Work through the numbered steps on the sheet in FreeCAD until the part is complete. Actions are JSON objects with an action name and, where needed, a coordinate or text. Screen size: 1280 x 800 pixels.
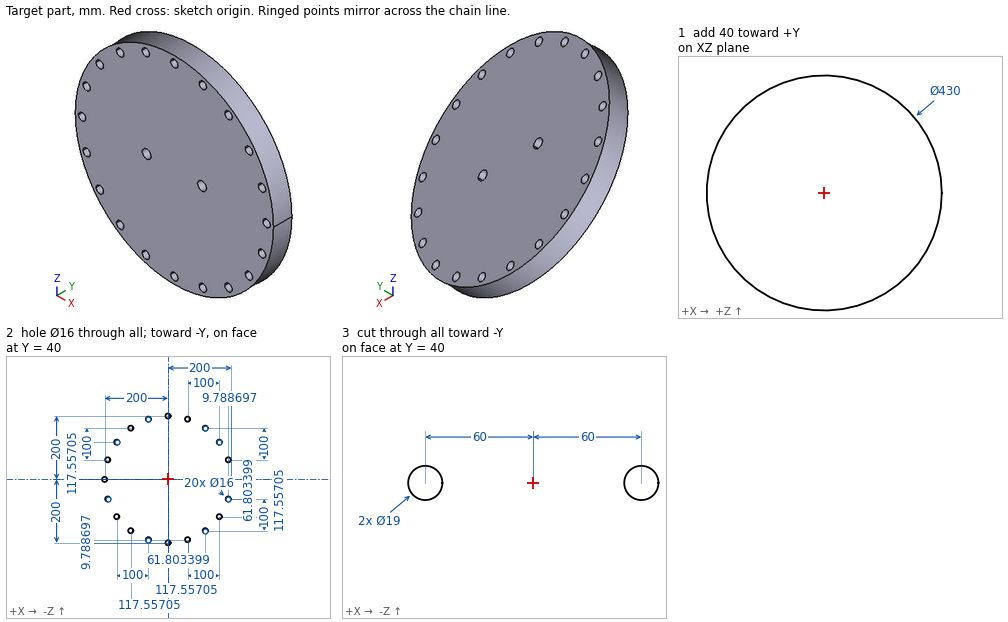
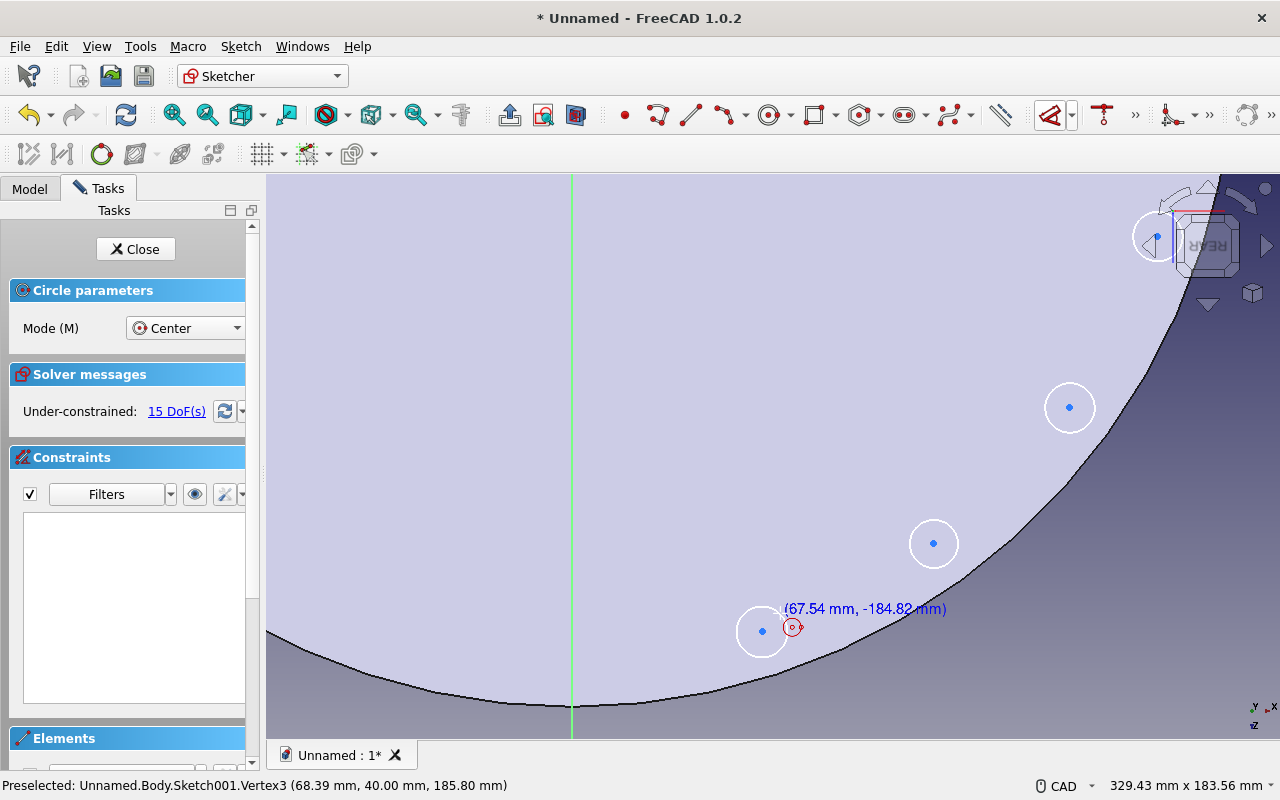
{"action": "left_click", "coordinate": [572, 661]}
{"action": "left_click", "coordinate": [590, 643]}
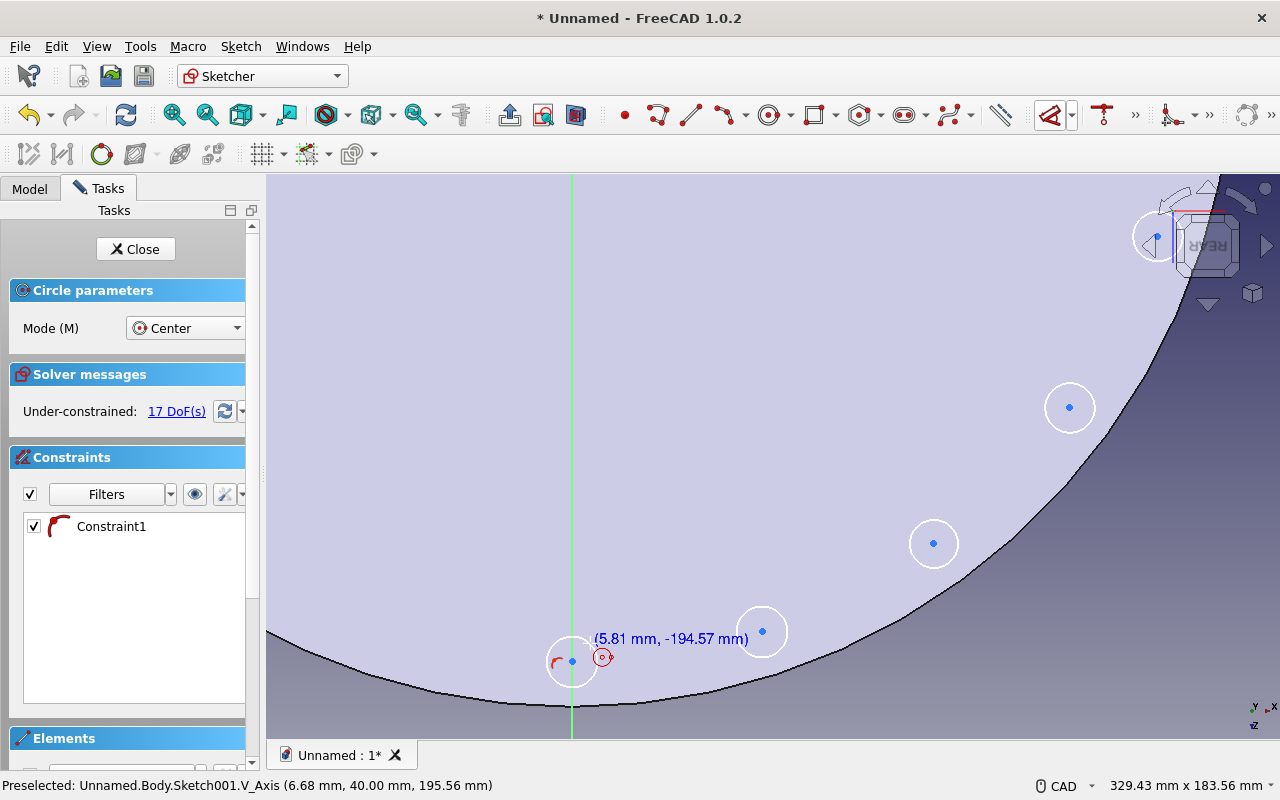
{"action": "left_click", "coordinate": [382, 631]}
{"action": "left_click", "coordinate": [399, 613]}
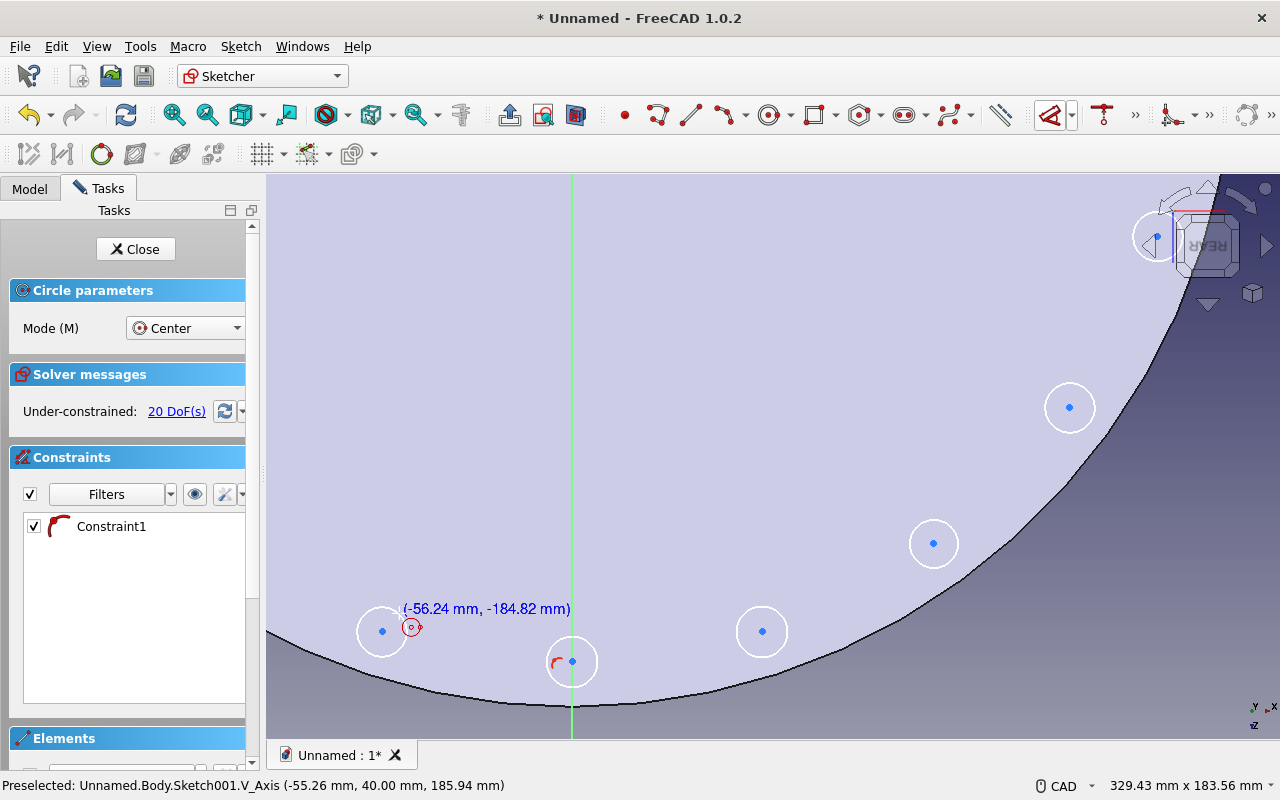
{"action": "scroll", "coordinate": [762, 634], "scroll_direction": "down", "scroll_amount": 6}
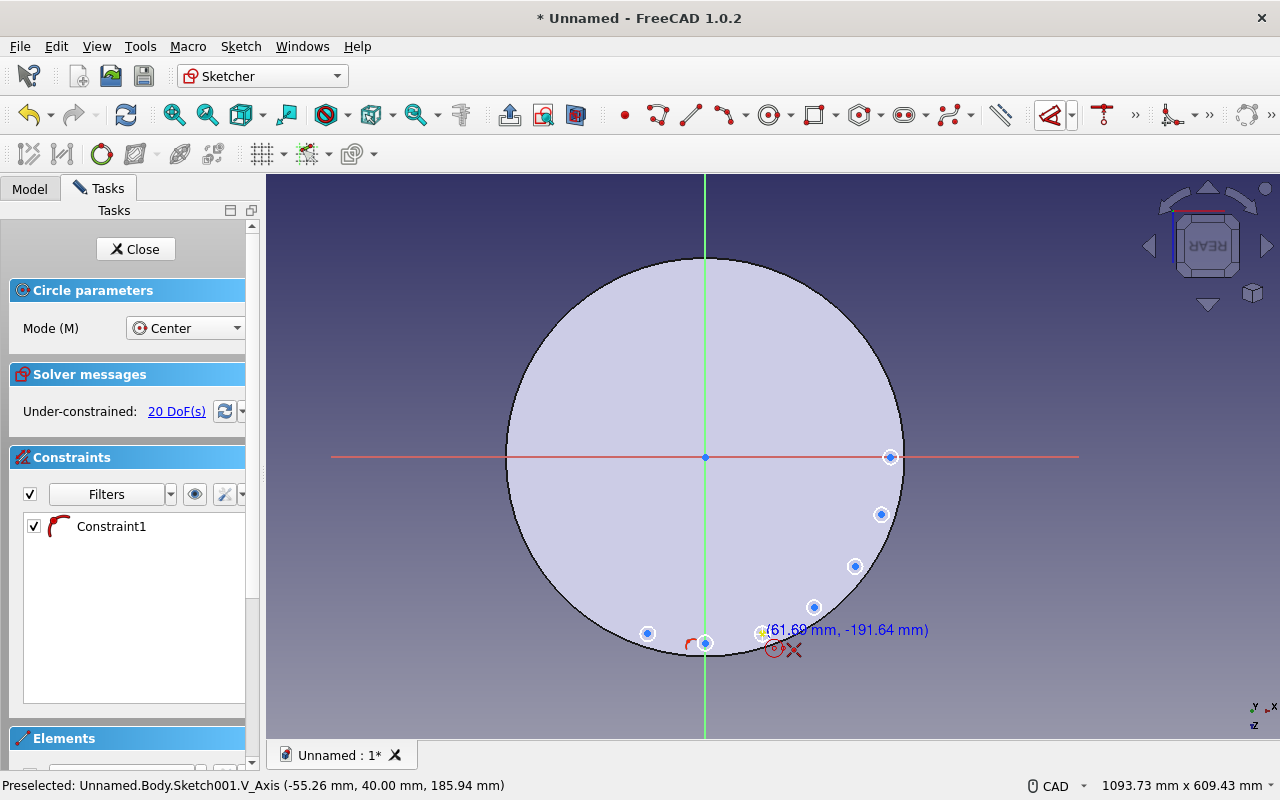
{"action": "scroll", "coordinate": [596, 607], "scroll_direction": "up", "scroll_amount": 6}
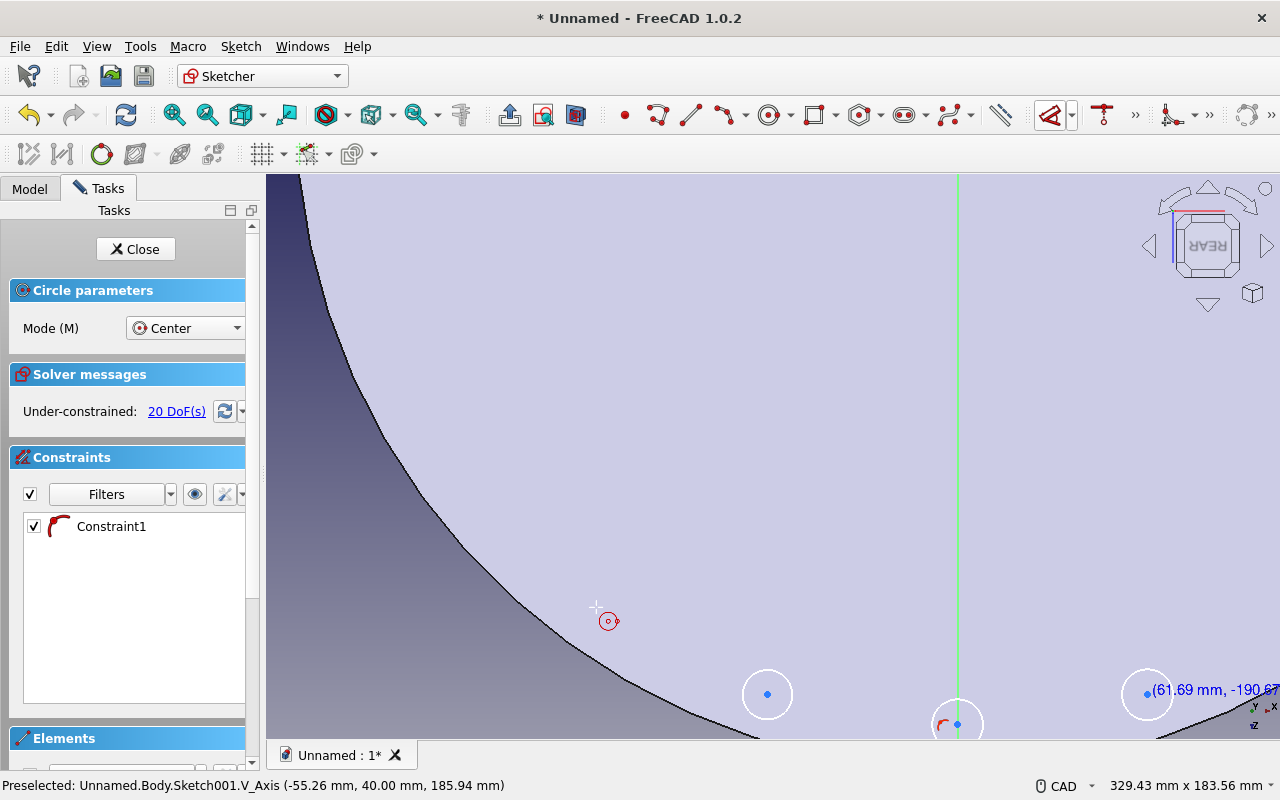
{"action": "left_click", "coordinate": [596, 606]}
{"action": "left_click", "coordinate": [613, 588]}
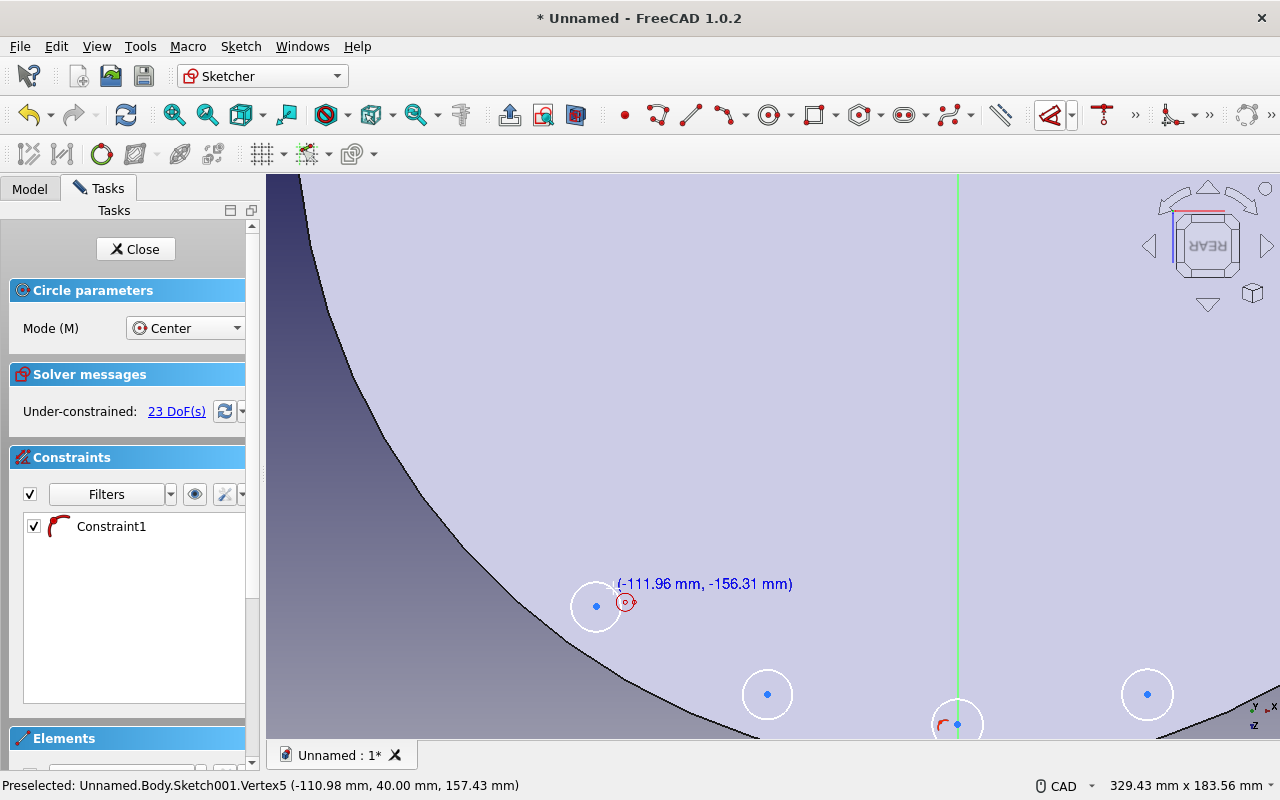
{"action": "left_click", "coordinate": [460, 470]}
{"action": "left_click", "coordinate": [477, 452]}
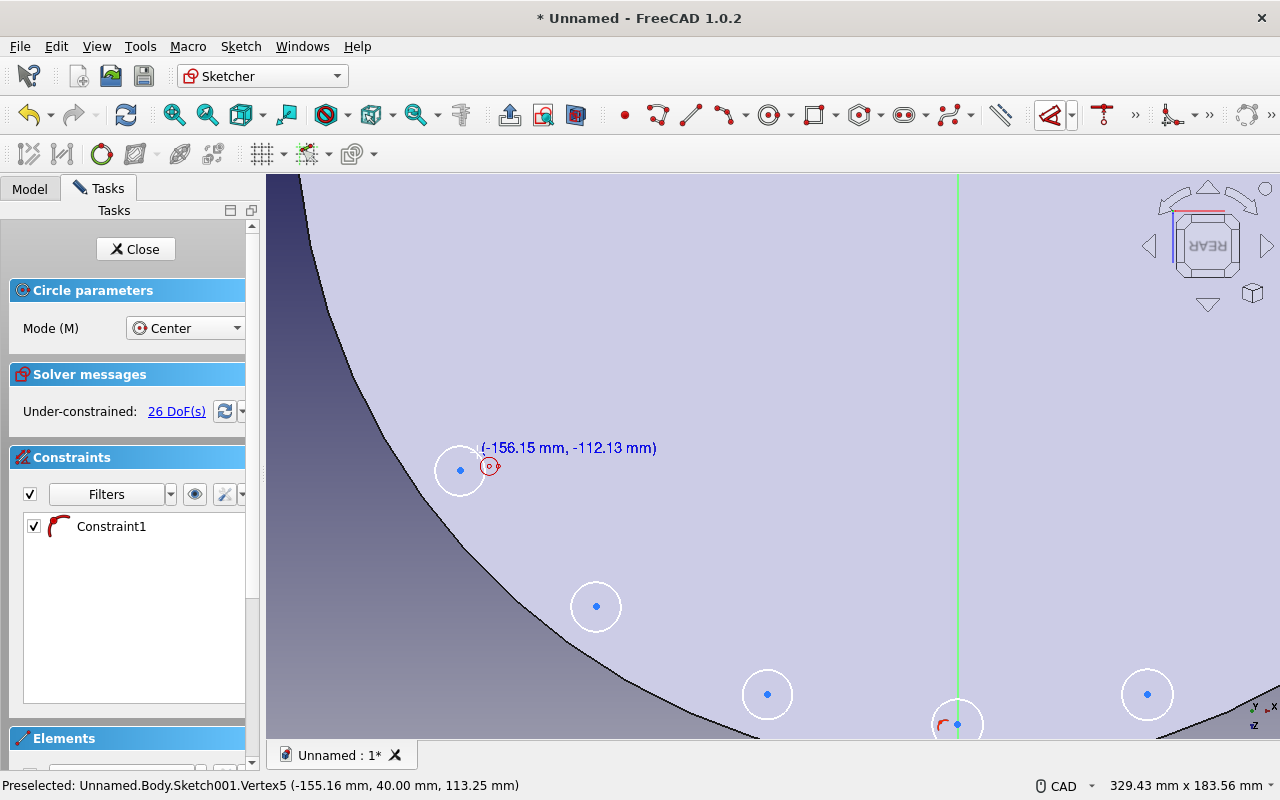
{"action": "left_click", "coordinate": [372, 298]}
{"action": "left_click", "coordinate": [390, 281]}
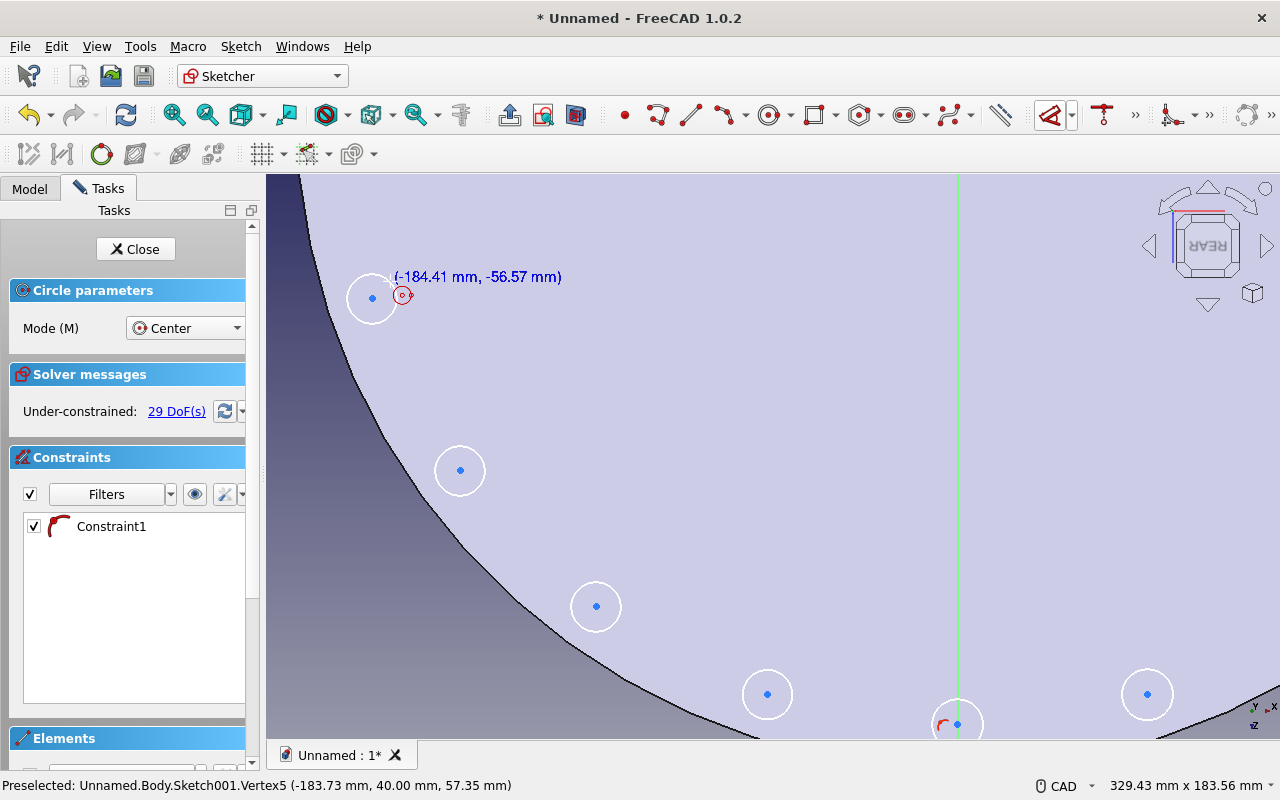
{"action": "scroll", "coordinate": [595, 607], "scroll_direction": "down", "scroll_amount": 6}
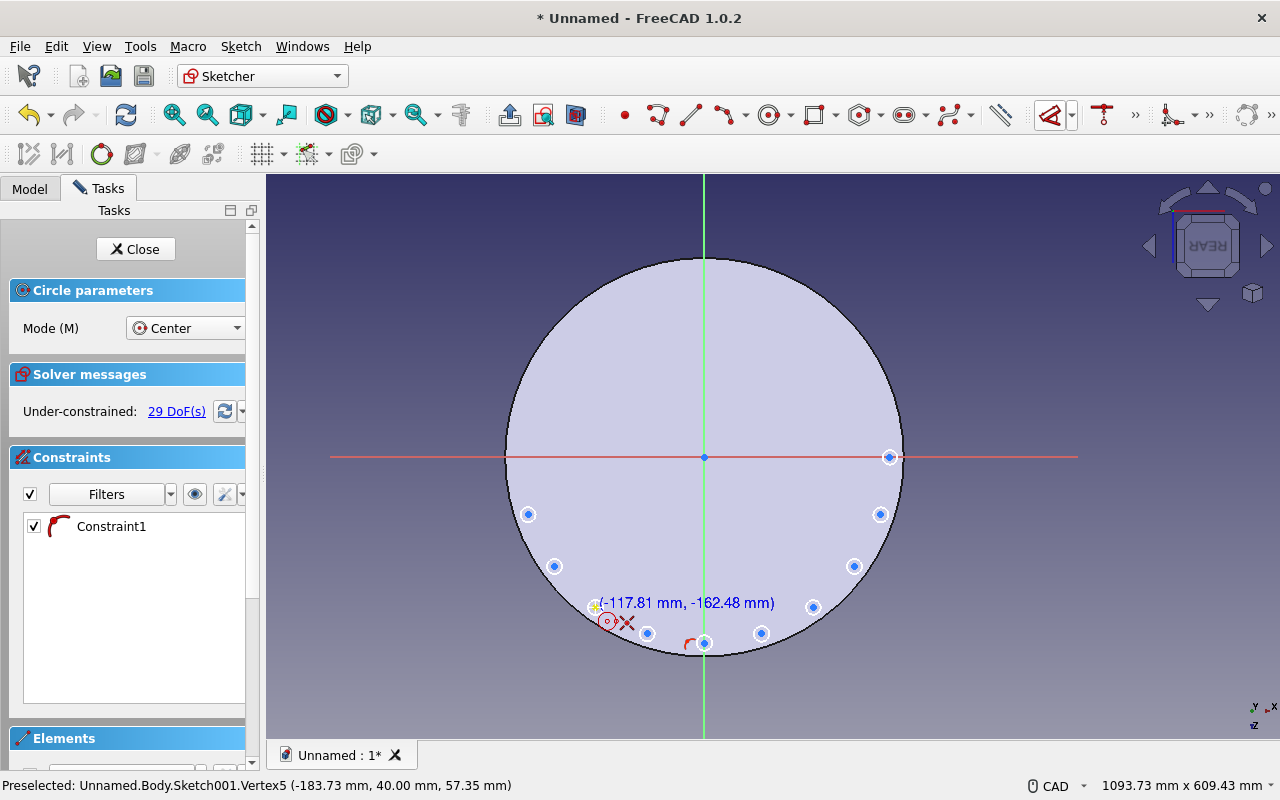
{"action": "scroll", "coordinate": [519, 457], "scroll_direction": "up", "scroll_amount": 6}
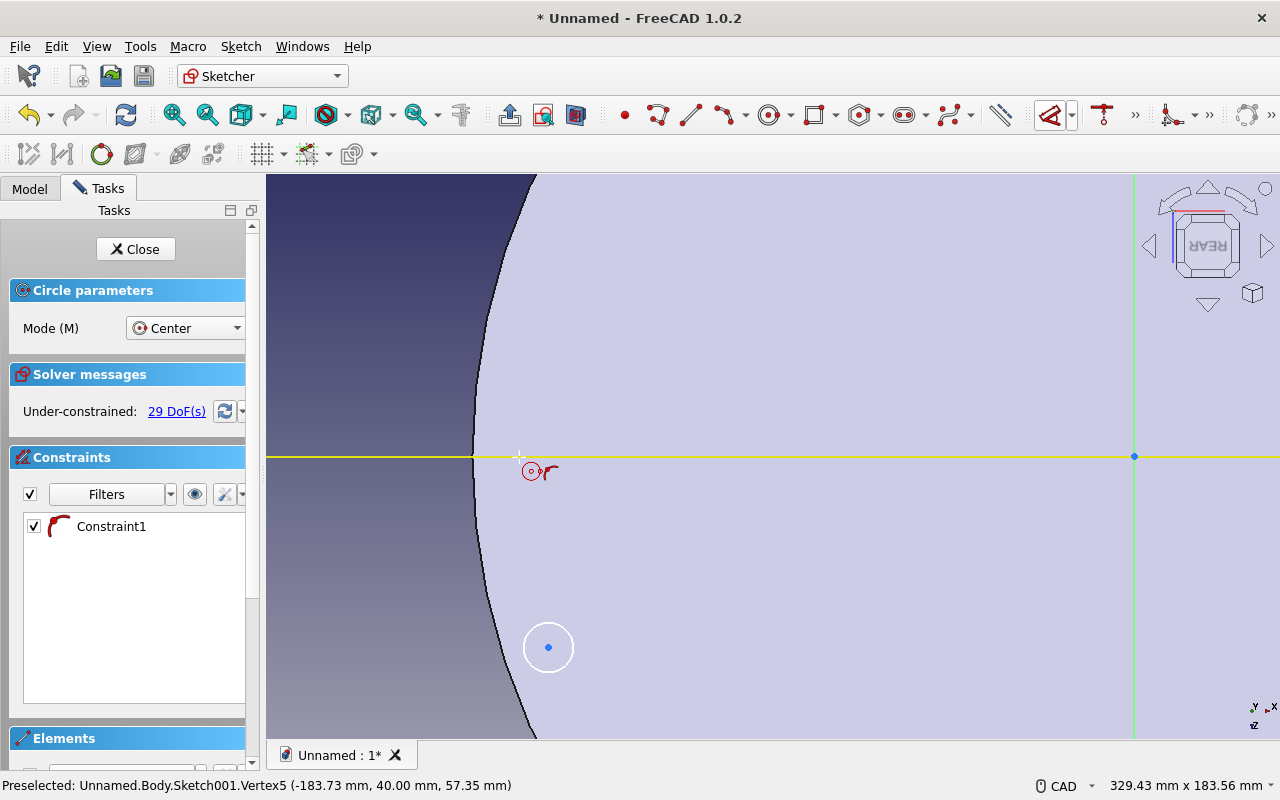
{"action": "left_click", "coordinate": [519, 457]}
{"action": "left_click", "coordinate": [536, 439]}